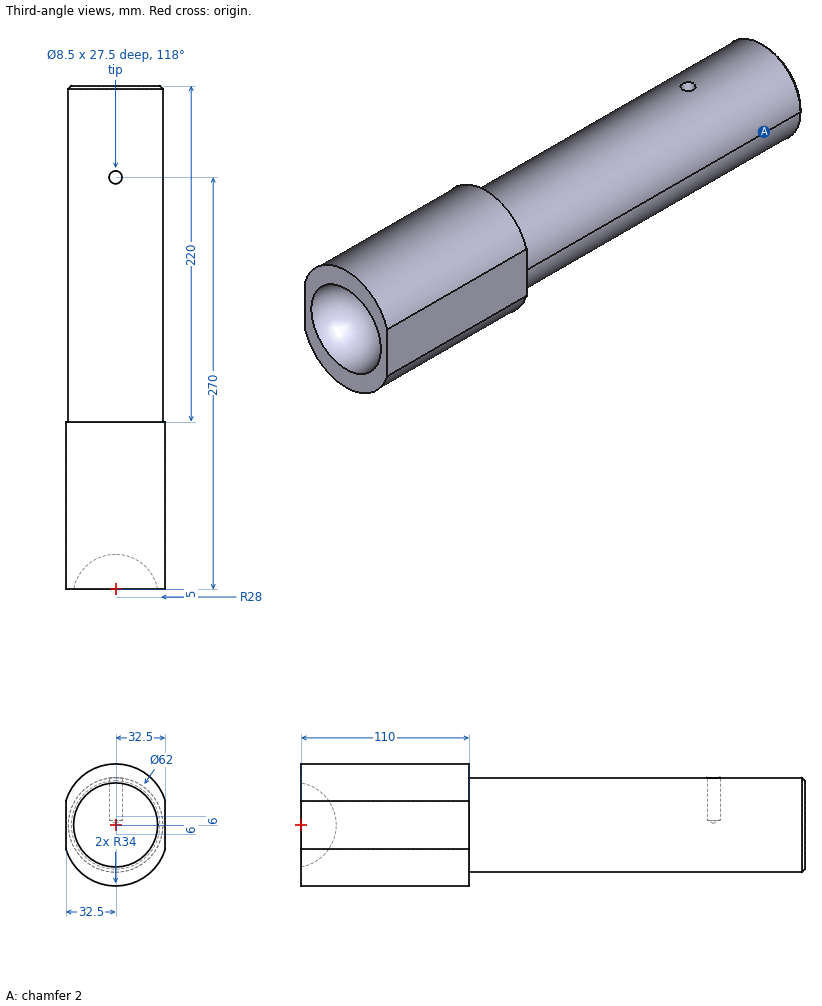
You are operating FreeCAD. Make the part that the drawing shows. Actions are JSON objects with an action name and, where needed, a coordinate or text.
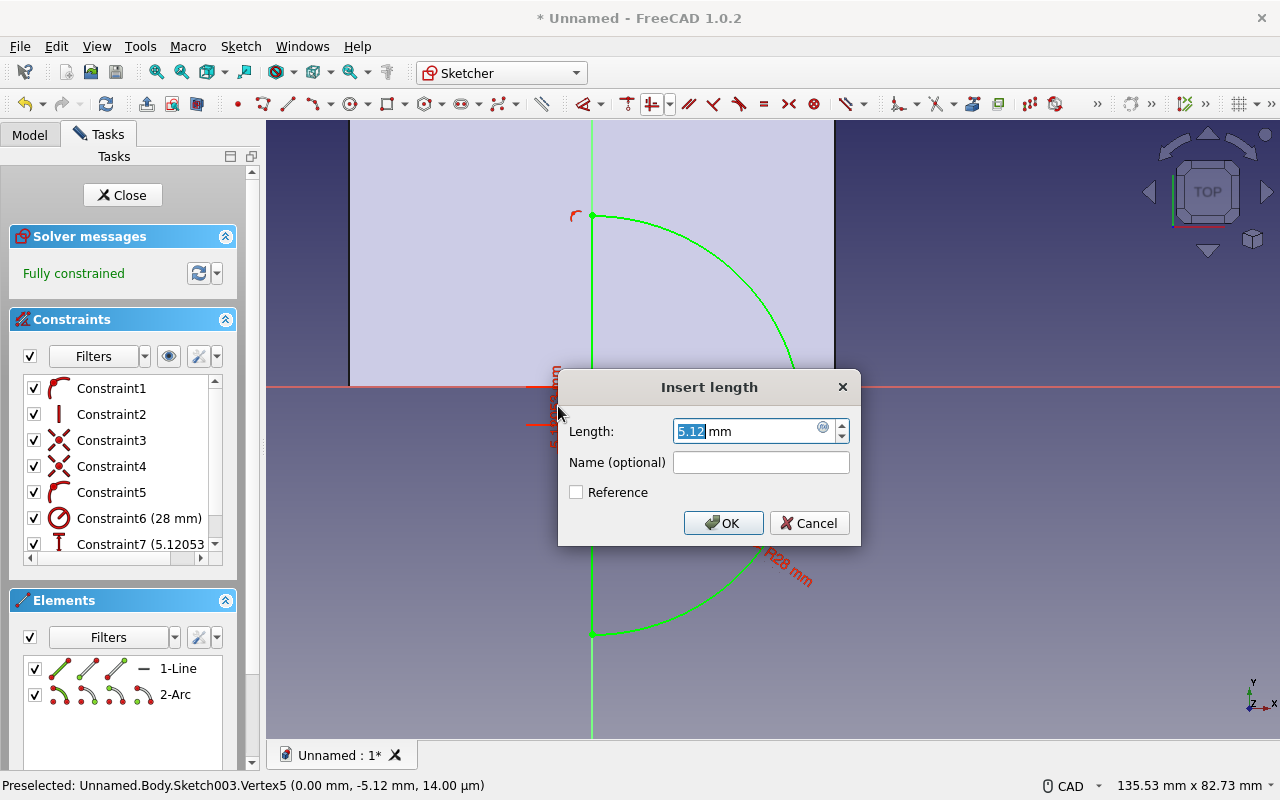
{"action": "type", "text": "5"}
{"action": "key", "text": "Return"}
{"action": "key", "text": "Escape"}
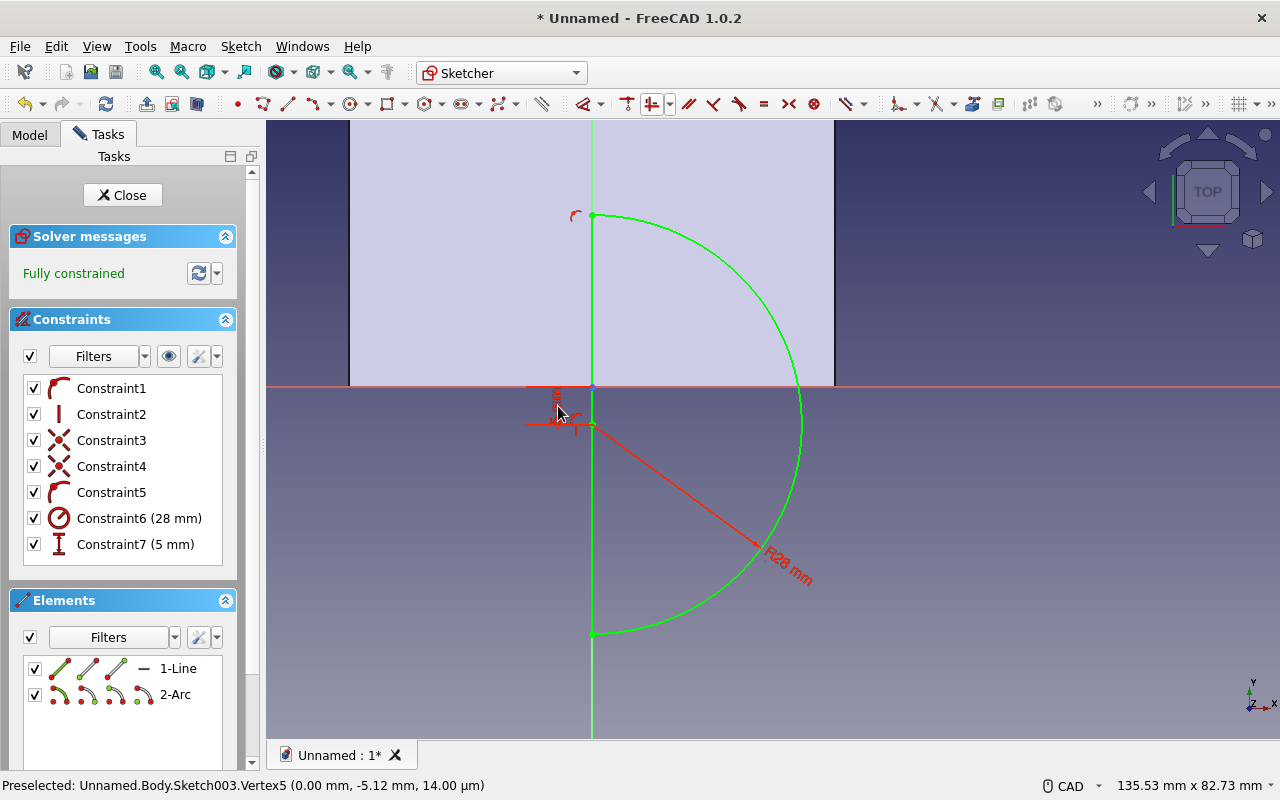
{"action": "left_click", "coordinate": [123, 195]}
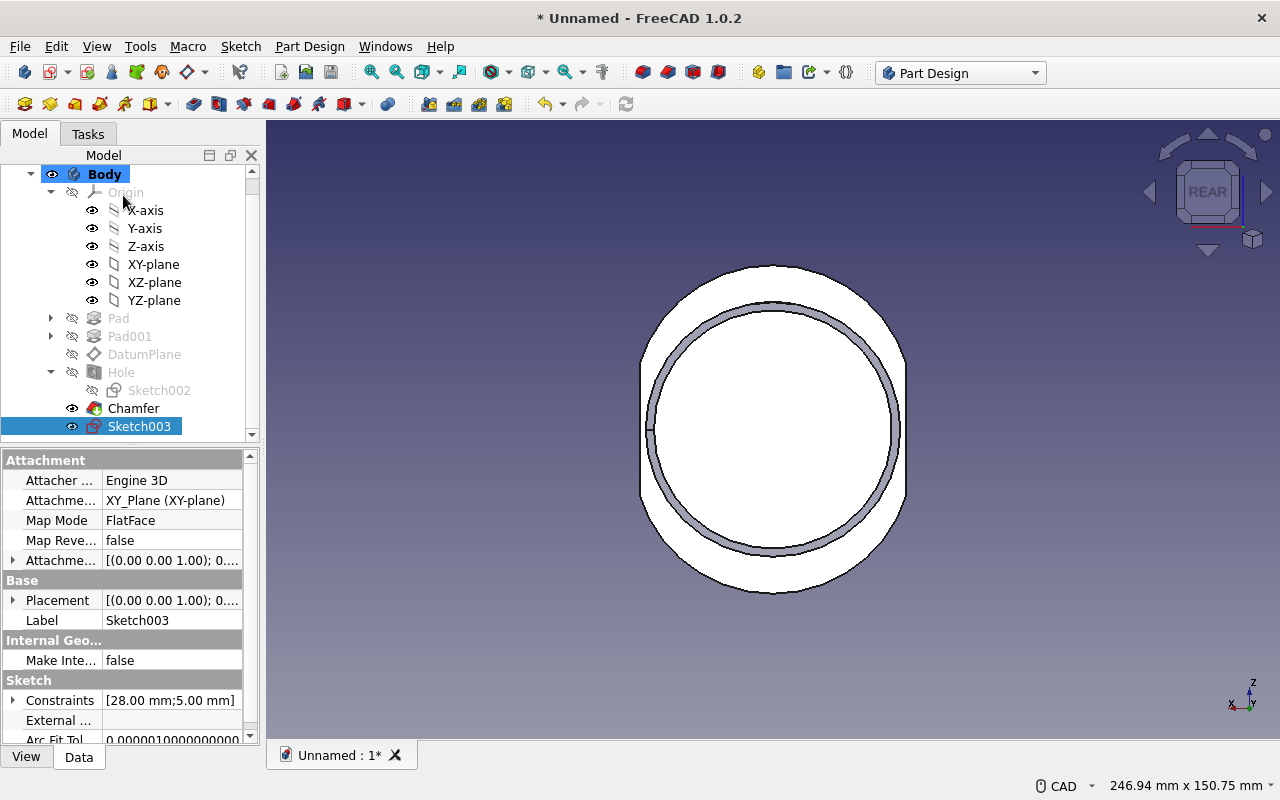
{"action": "left_click", "coordinate": [244, 104]}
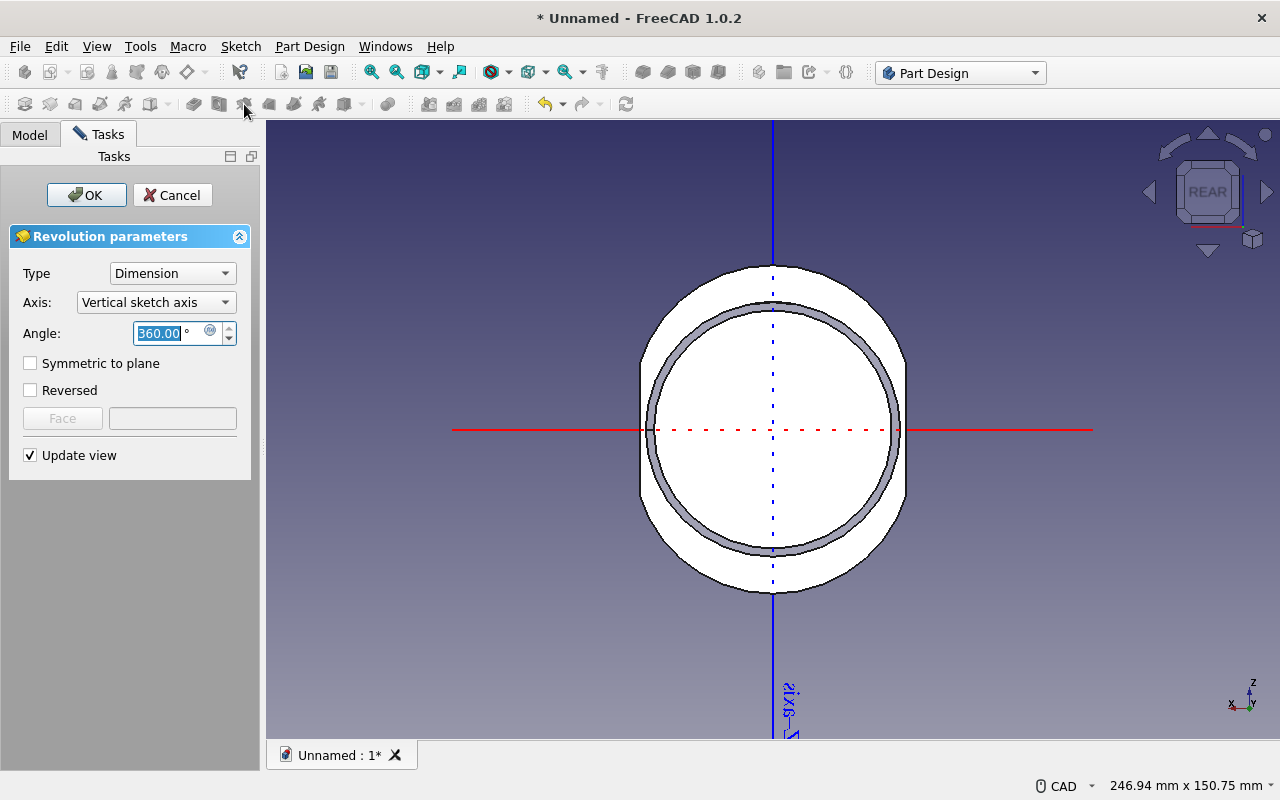
{"action": "left_click", "coordinate": [87, 195]}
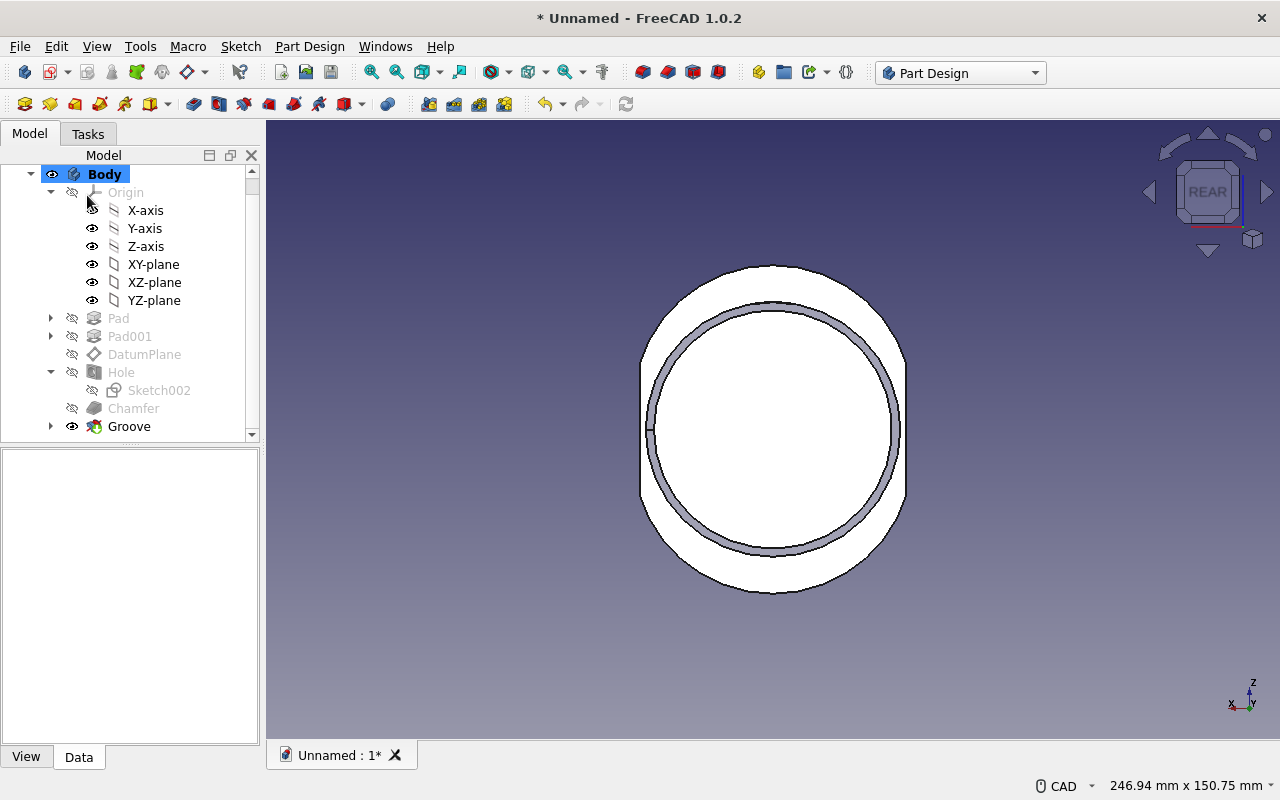
{"action": "key", "text": "0"}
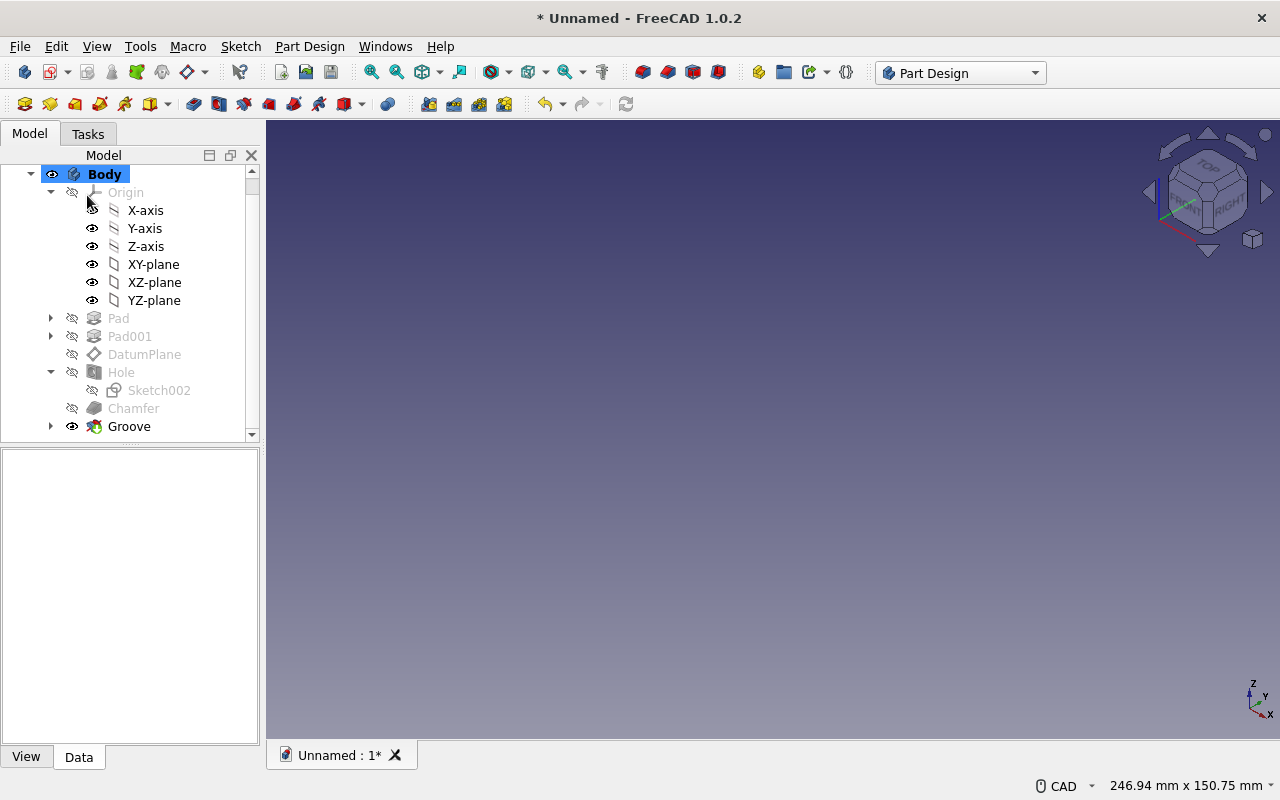
{"action": "left_click", "coordinate": [372, 72]}